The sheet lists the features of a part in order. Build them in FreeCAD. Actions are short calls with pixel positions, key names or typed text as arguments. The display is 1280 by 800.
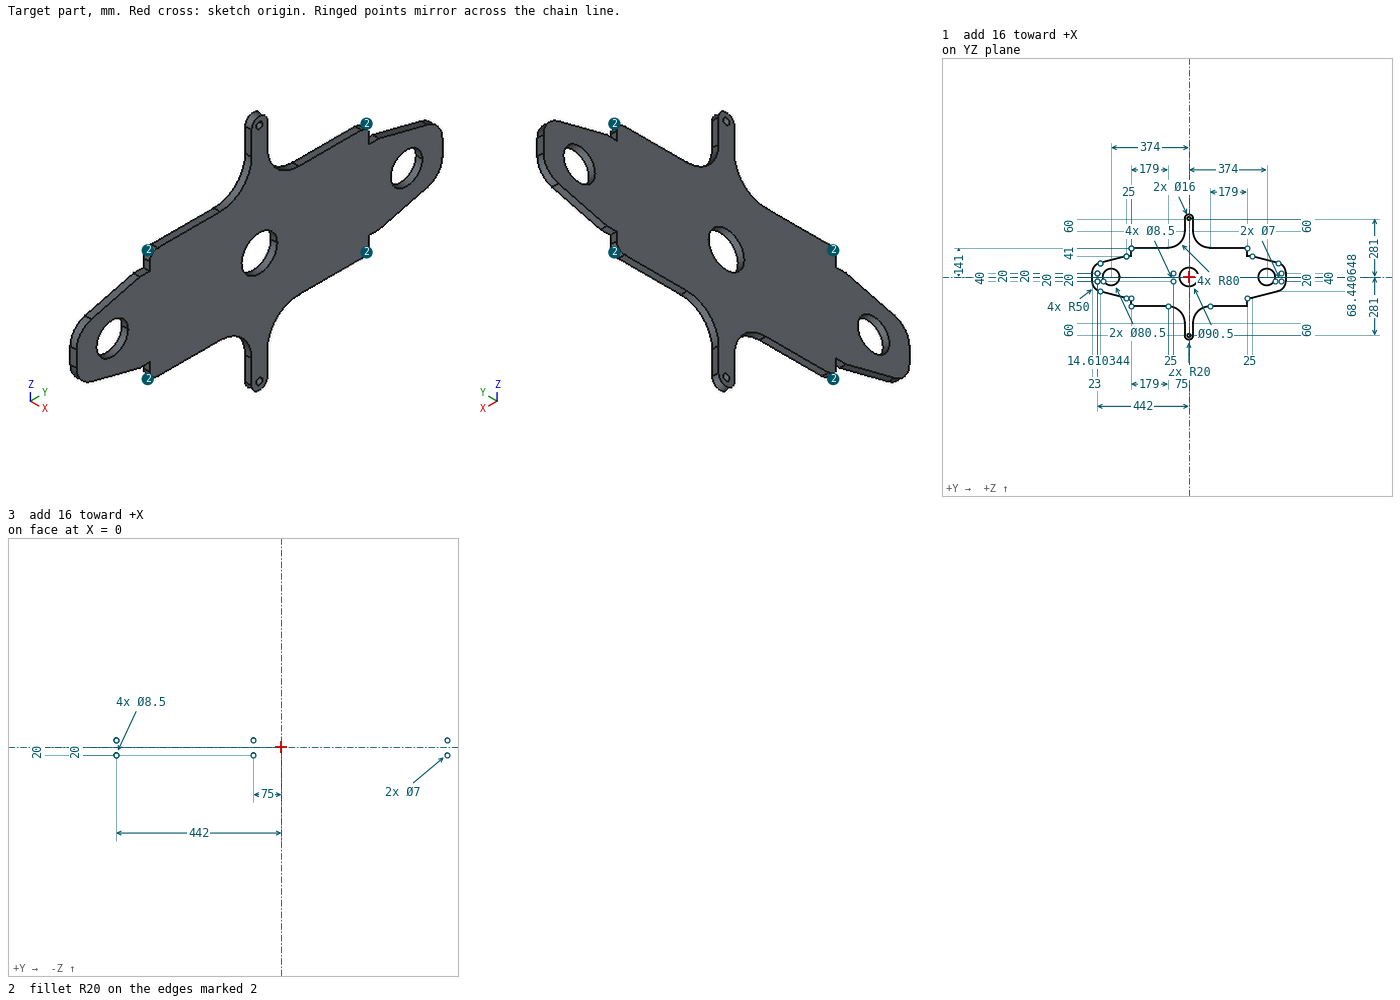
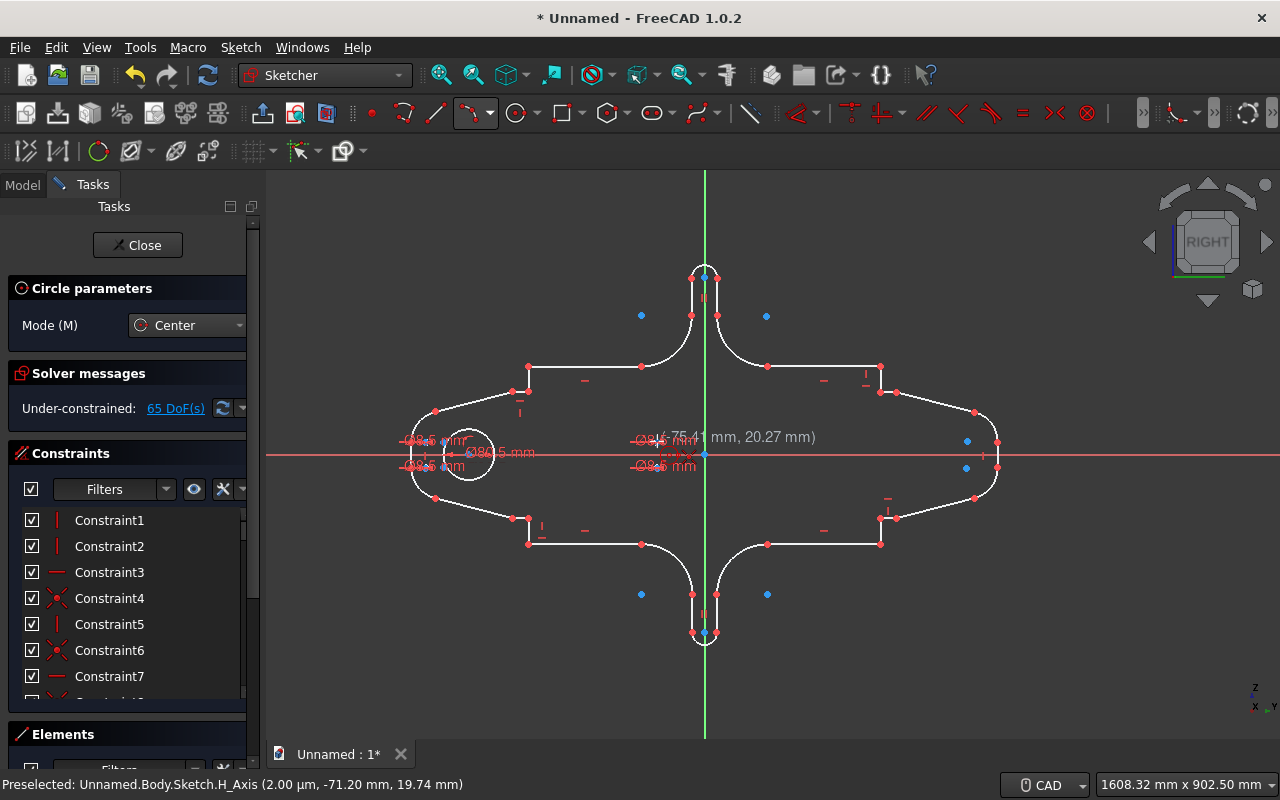
scroll(705, 632, up, 8)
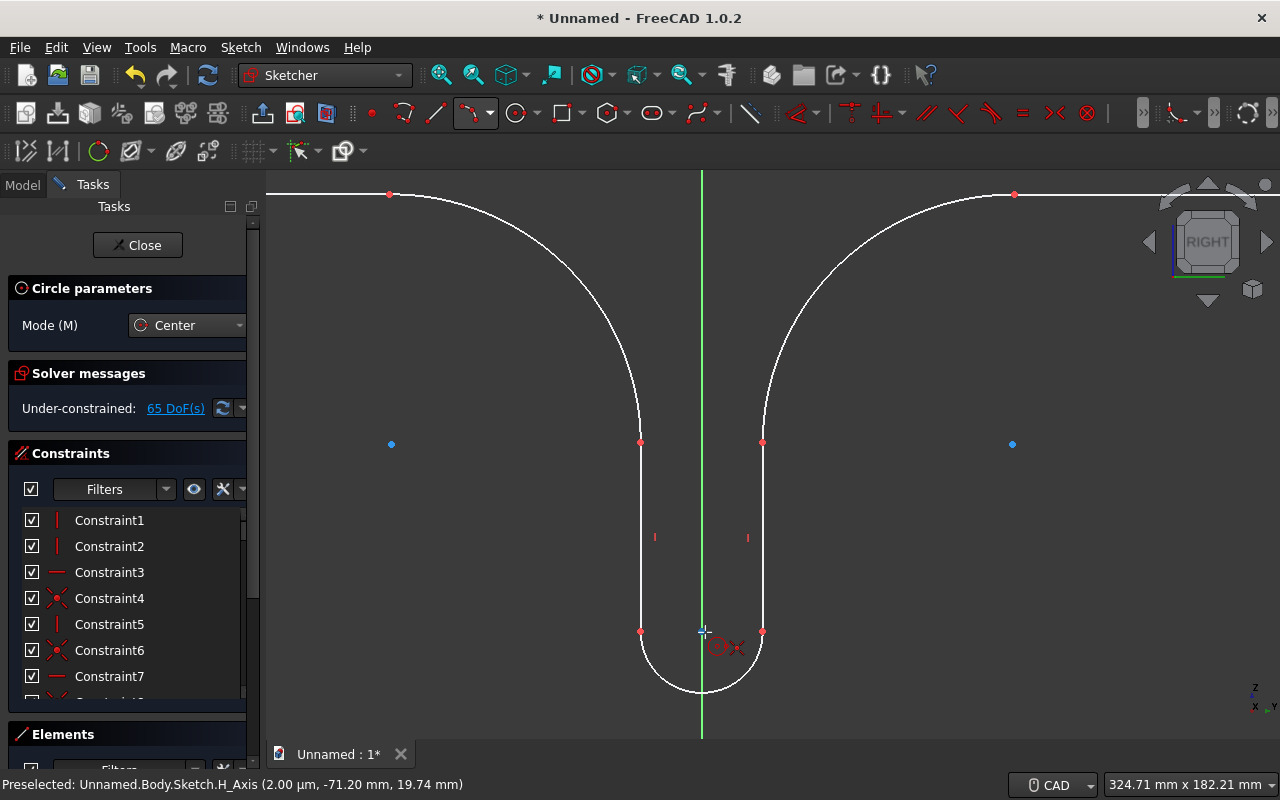
scroll(705, 633, down, 8)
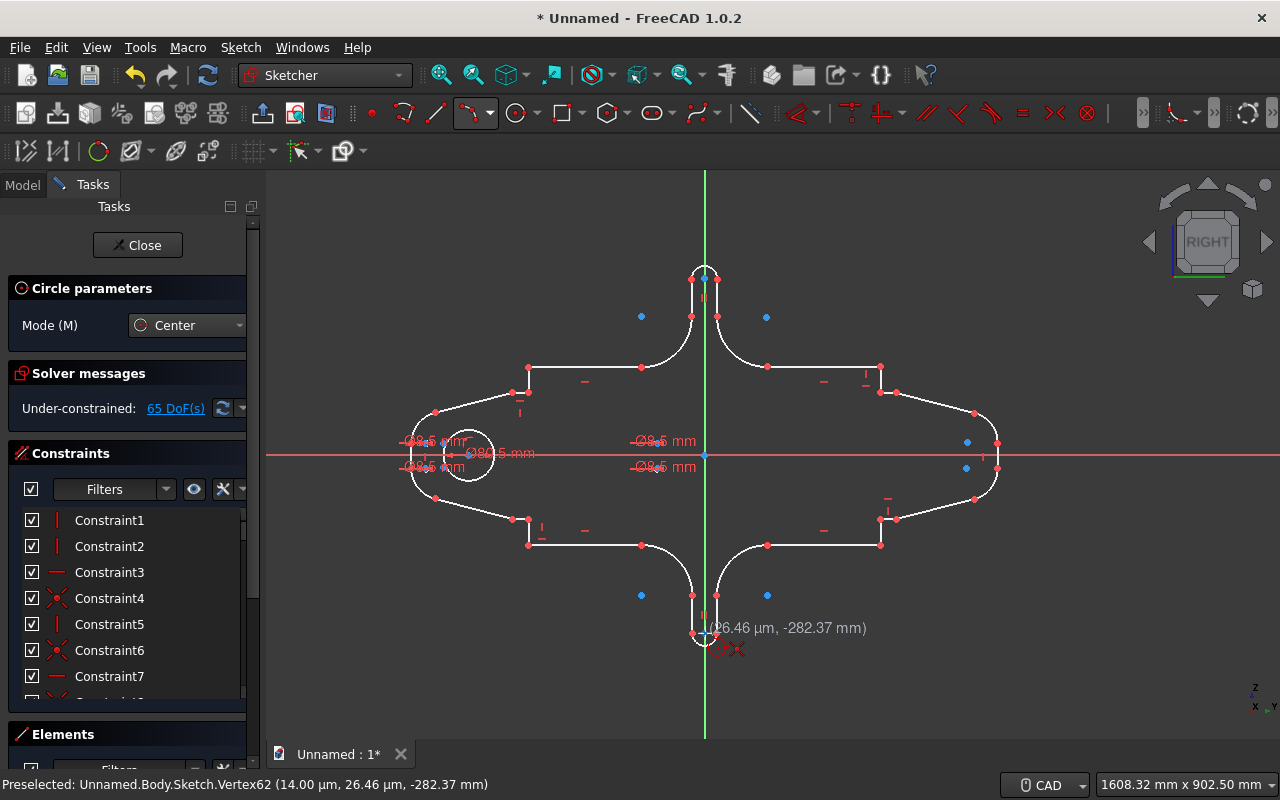
scroll(705, 633, up, 2)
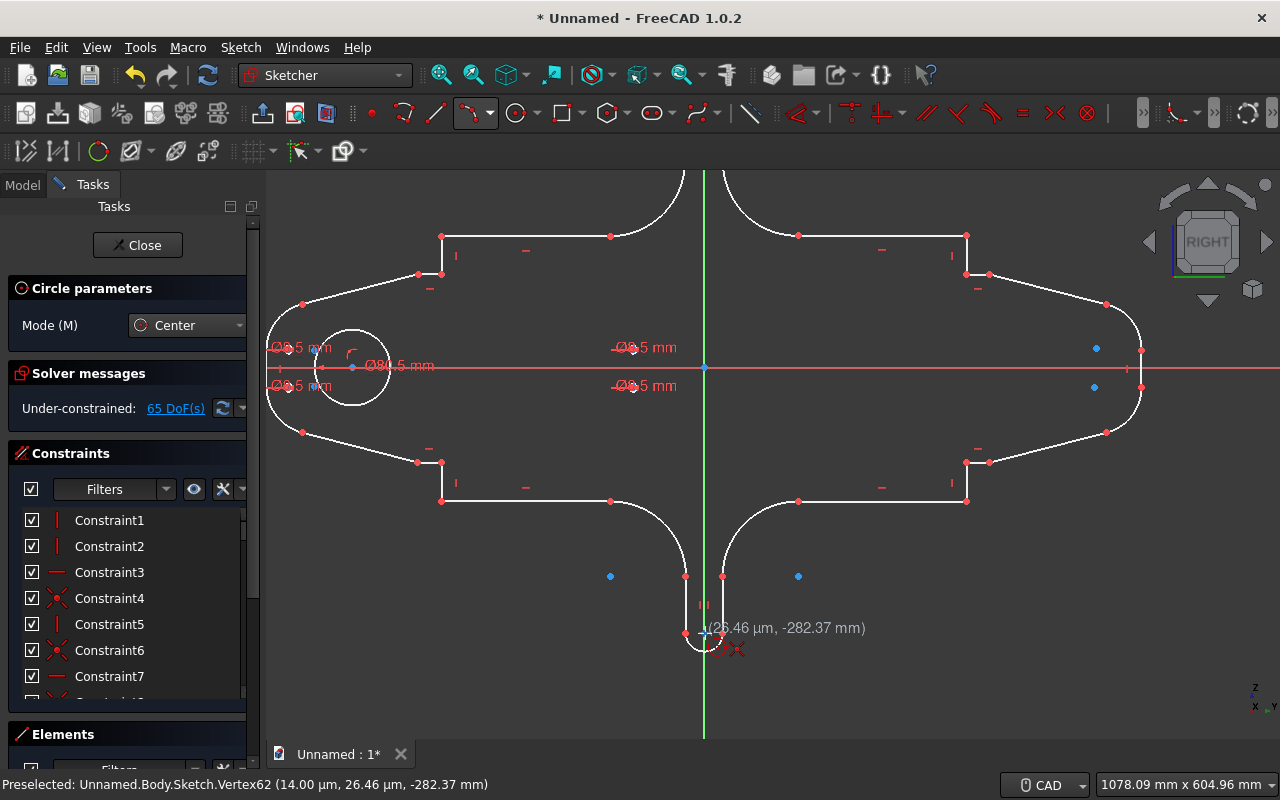
click(704, 632)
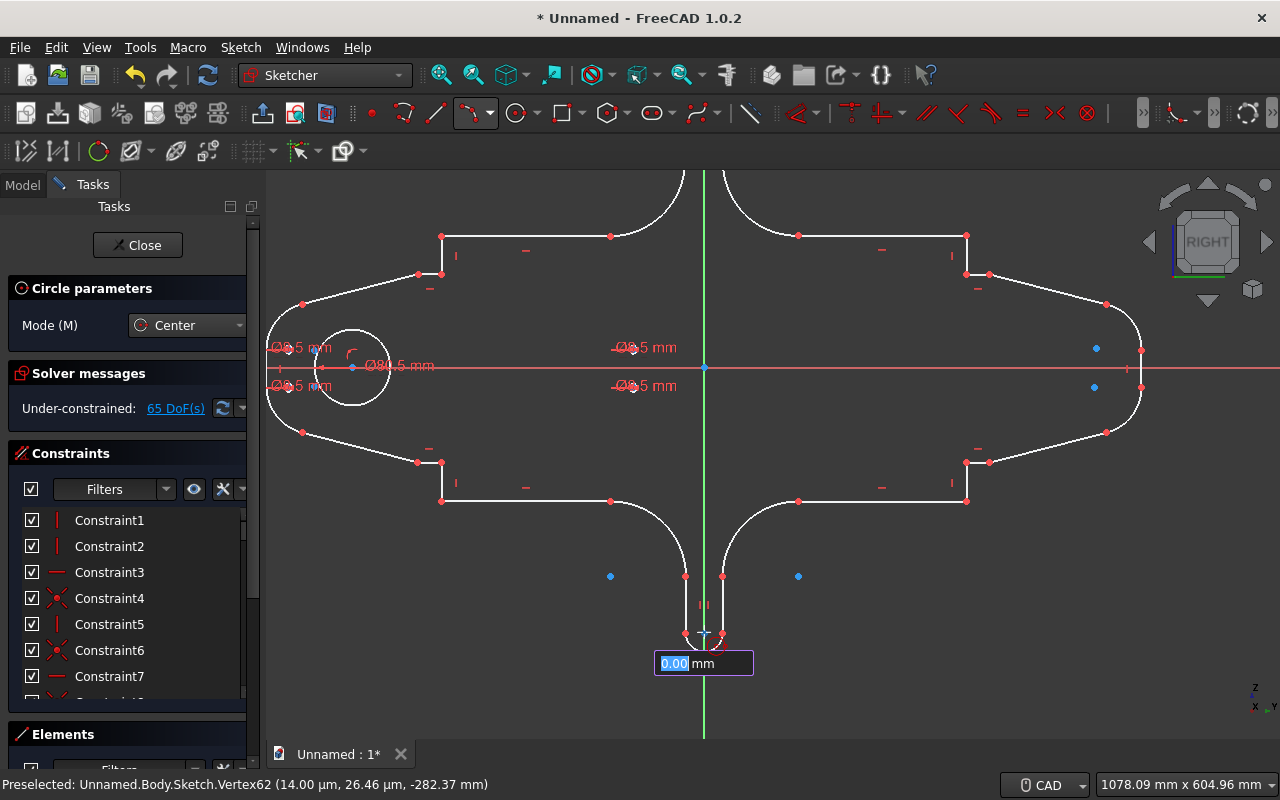
scroll(711, 629, up, 5)
move(711, 629)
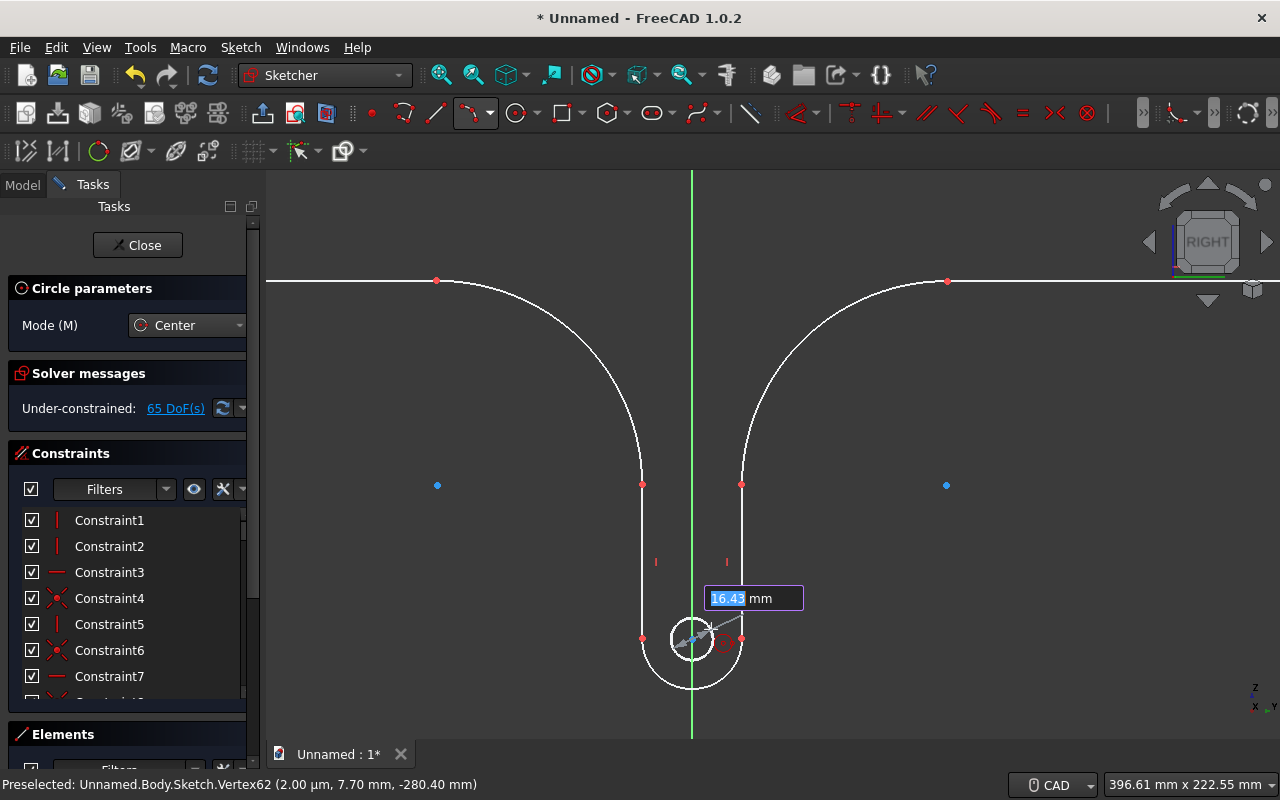
text(16)
key(Return)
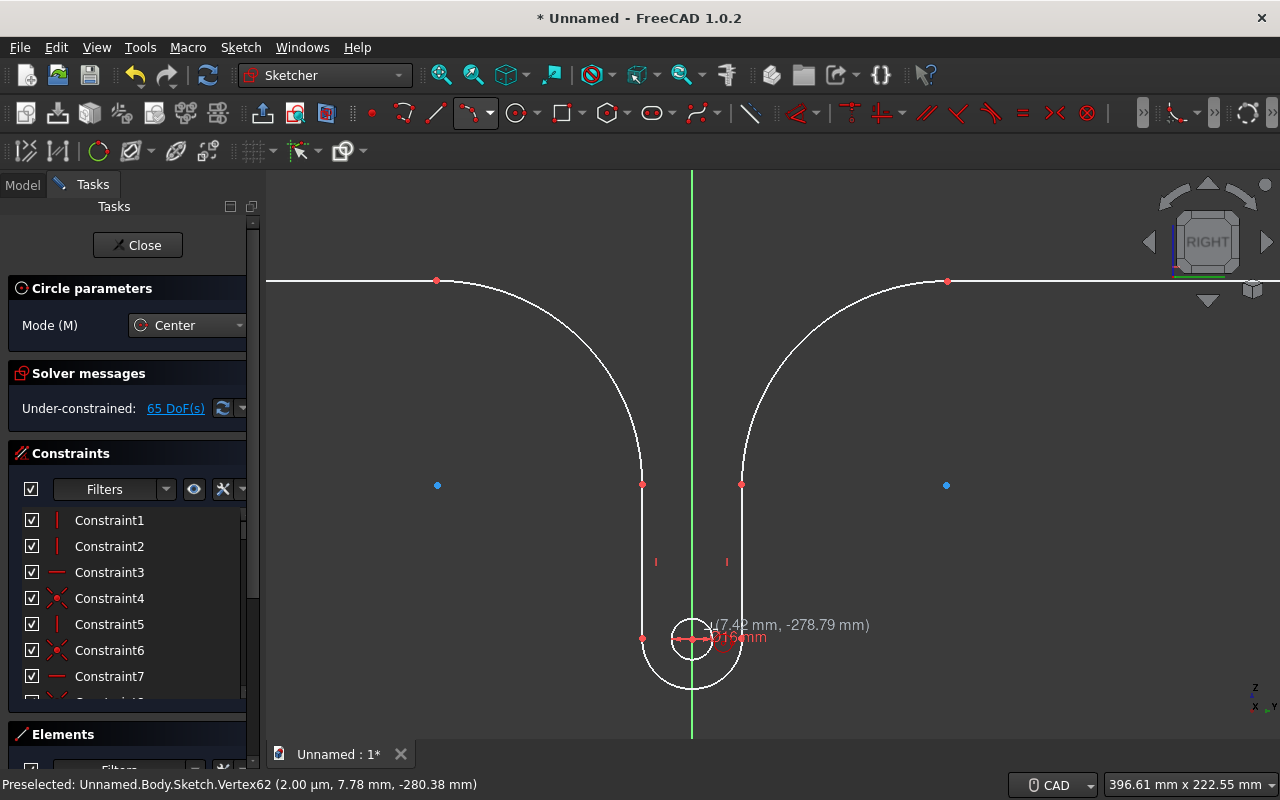
scroll(709, 630, down, 7)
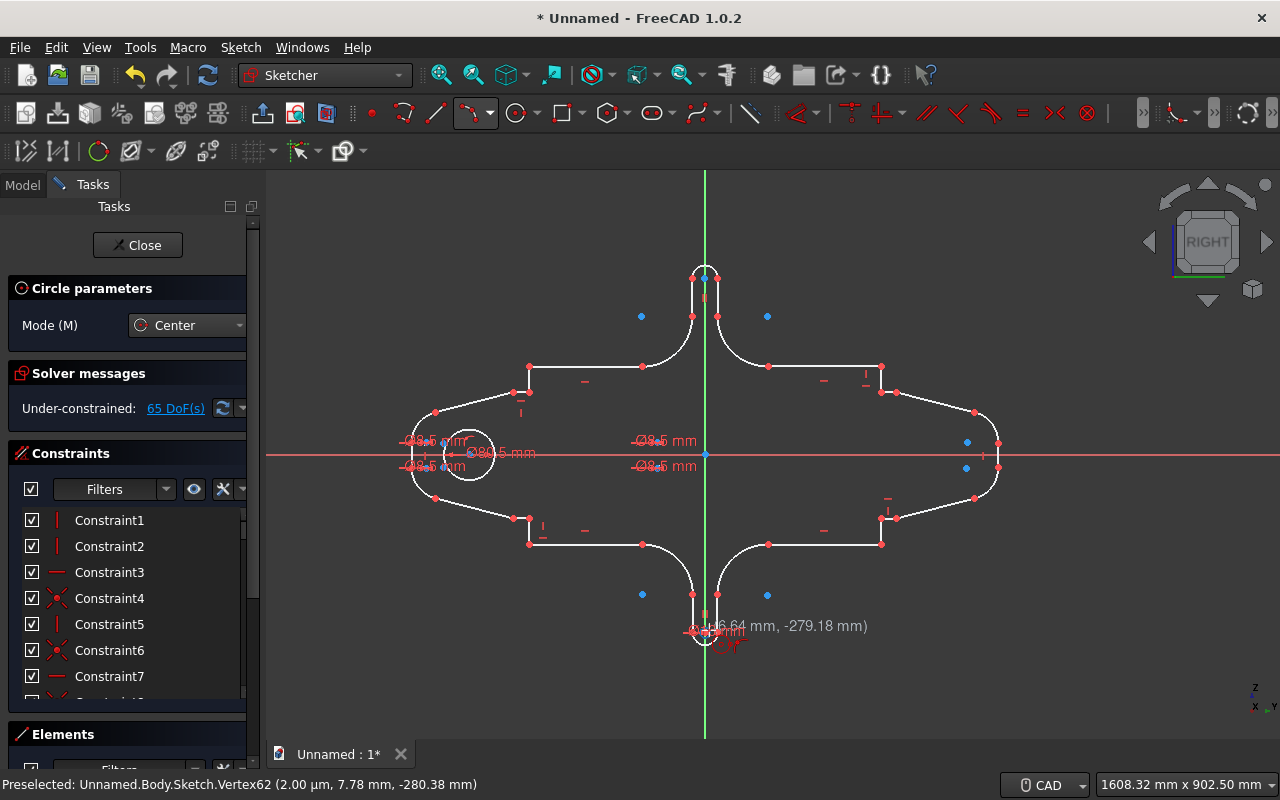
scroll(984, 467, up, 12)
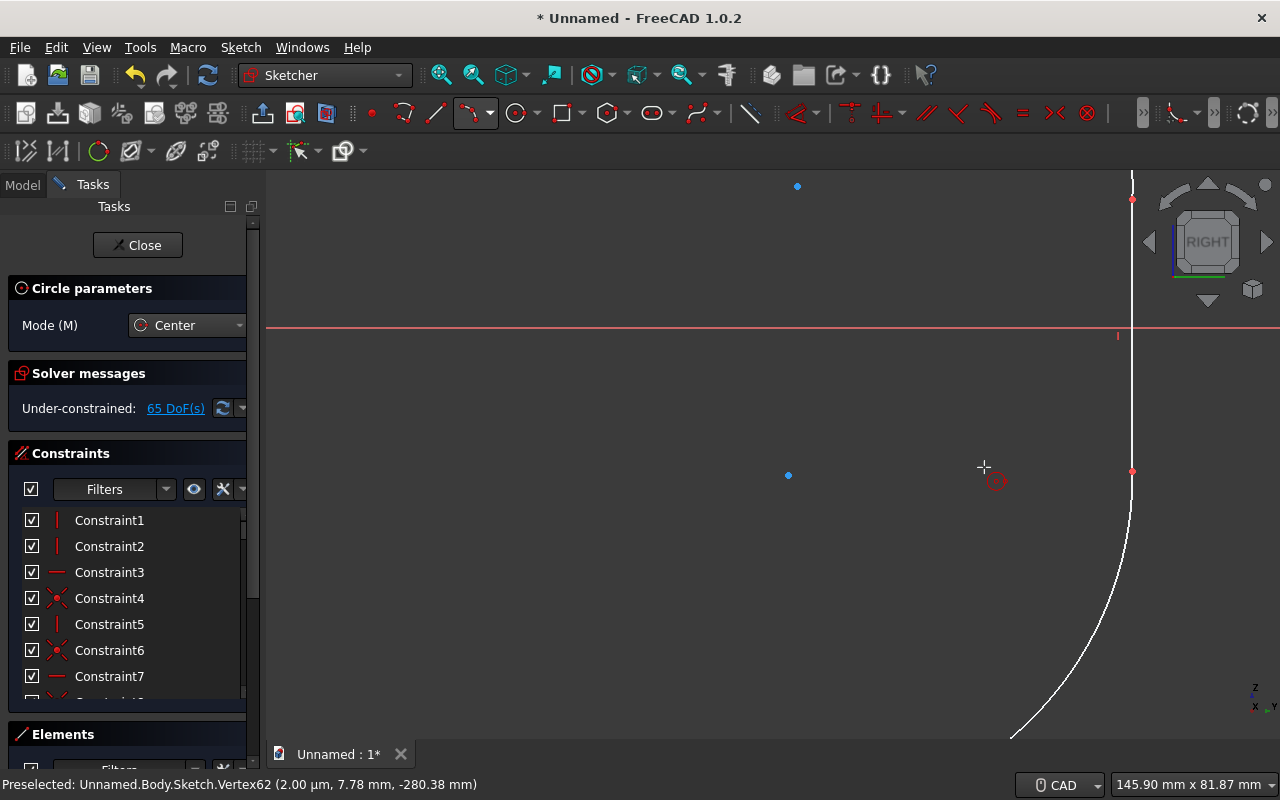
scroll(984, 467, down, 12)